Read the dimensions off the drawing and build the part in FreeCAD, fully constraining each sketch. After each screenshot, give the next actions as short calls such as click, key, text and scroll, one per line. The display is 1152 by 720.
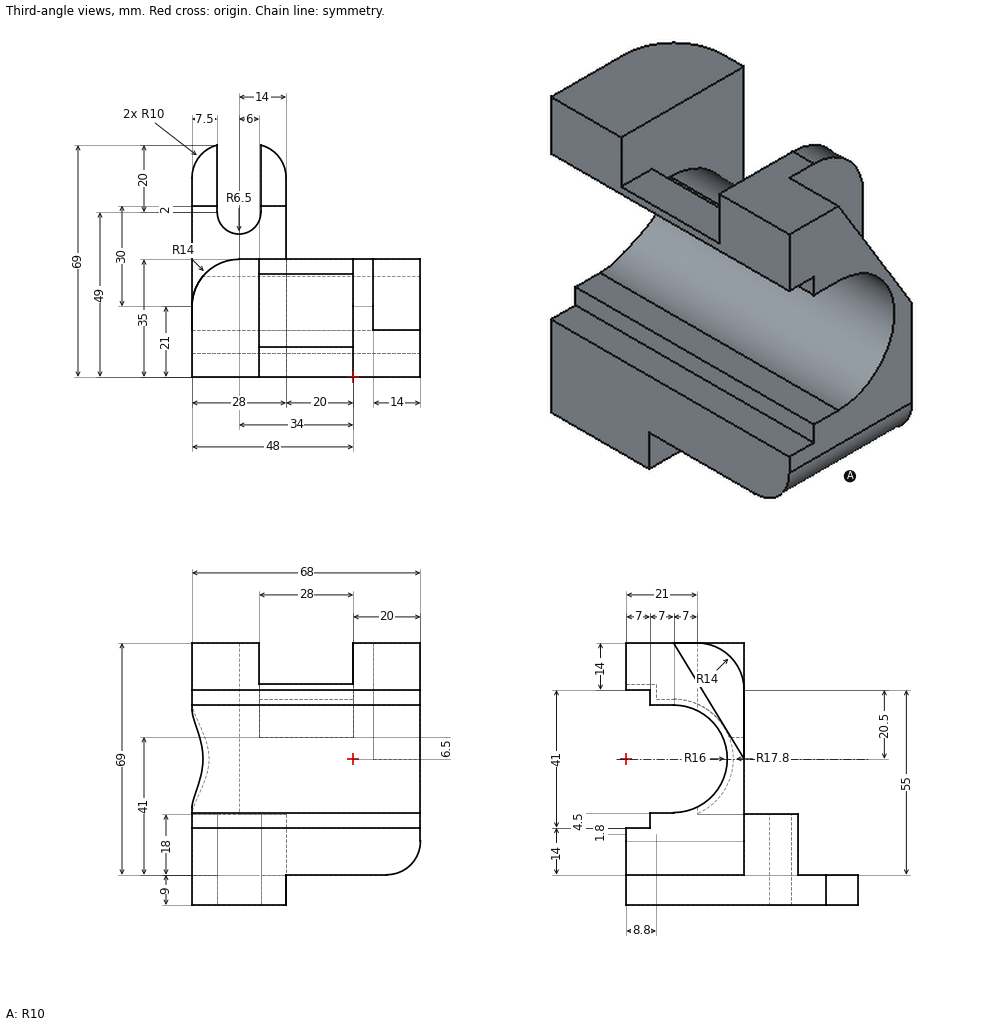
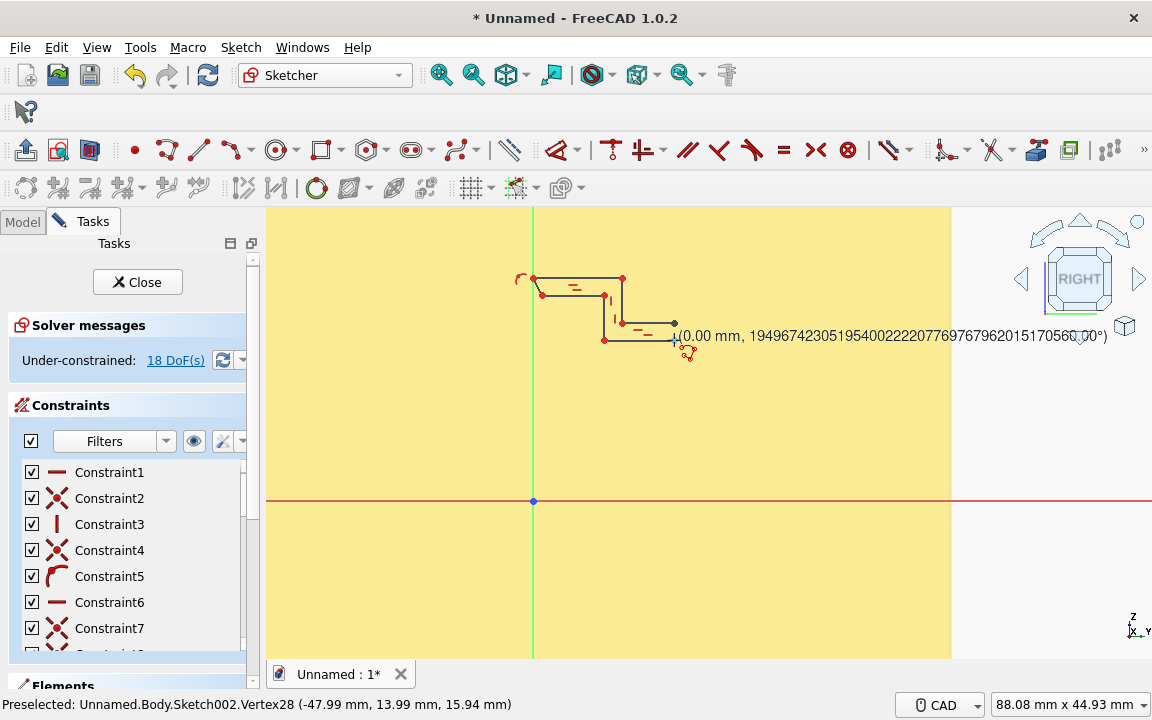
click(232, 150)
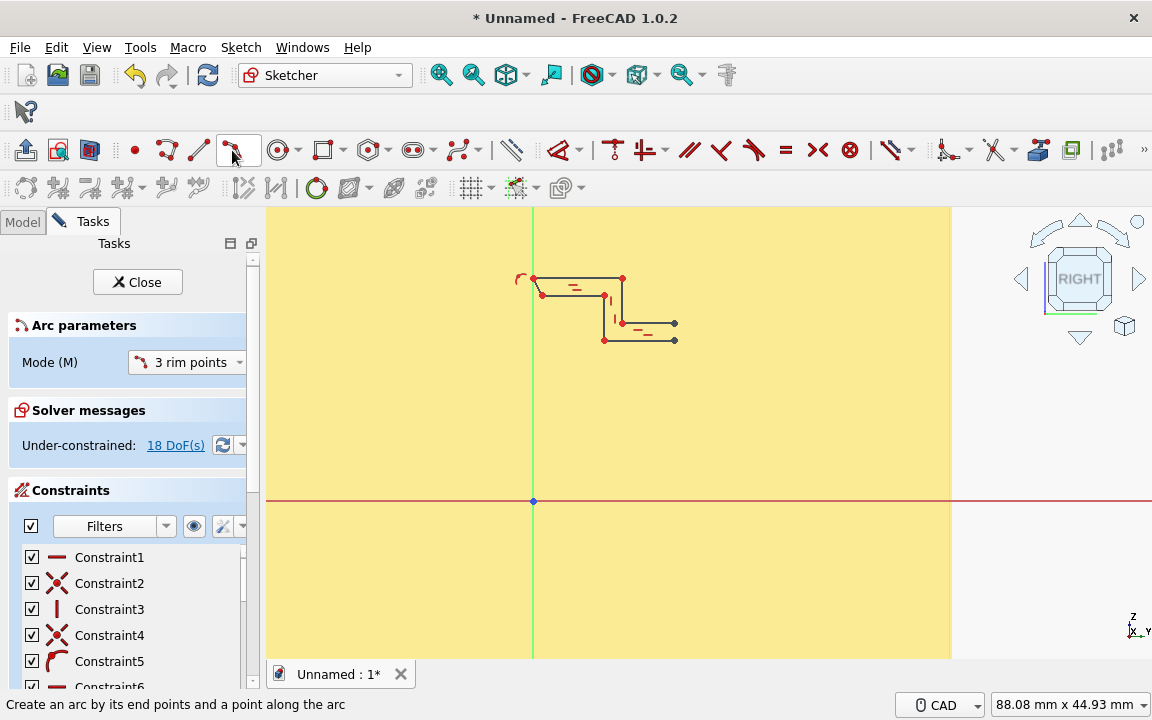
scroll(533, 294, down, 2)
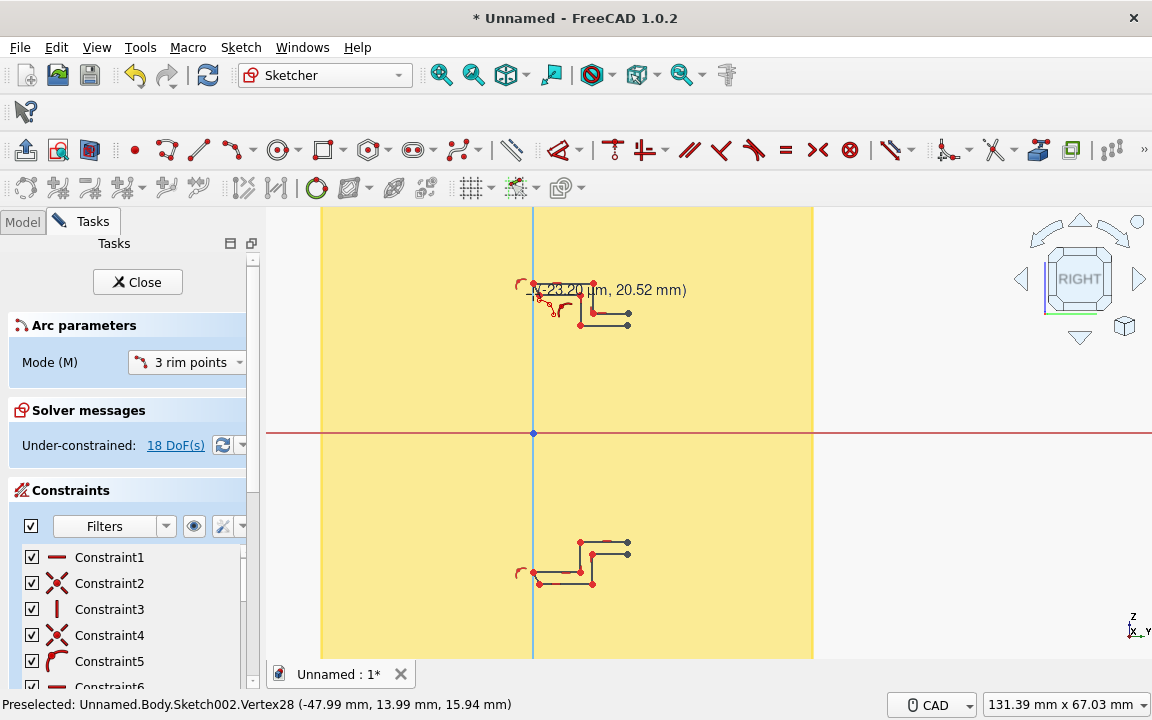
scroll(628, 553, up, 2)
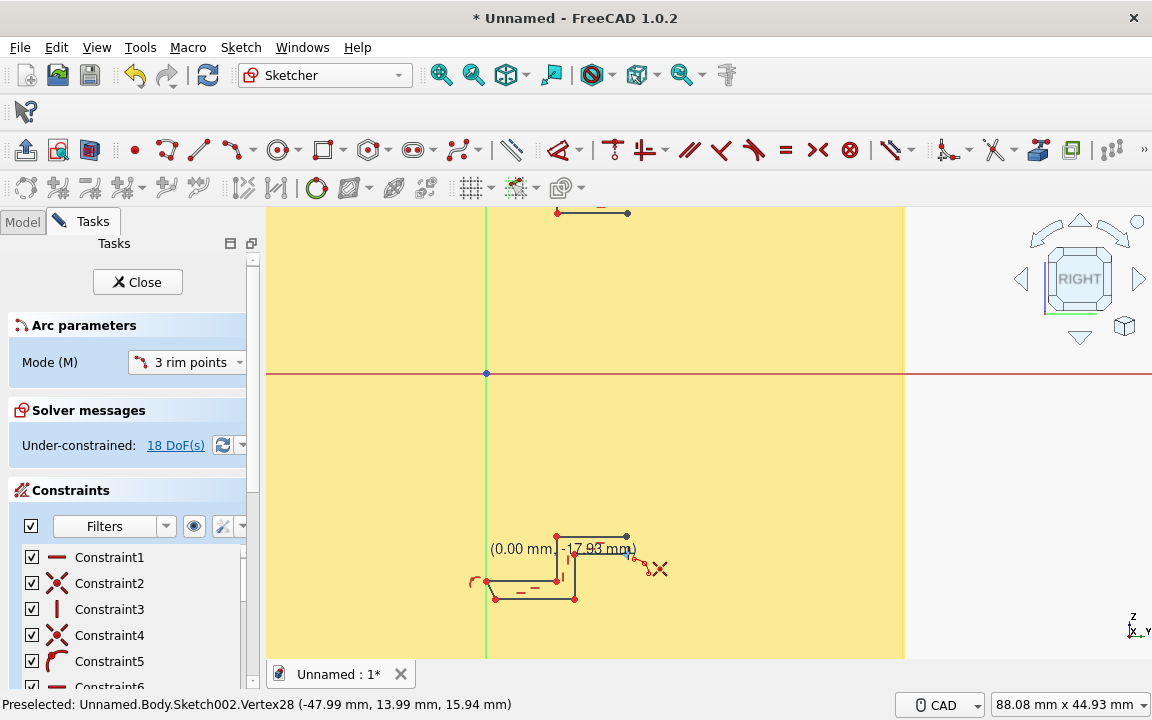
click(627, 554)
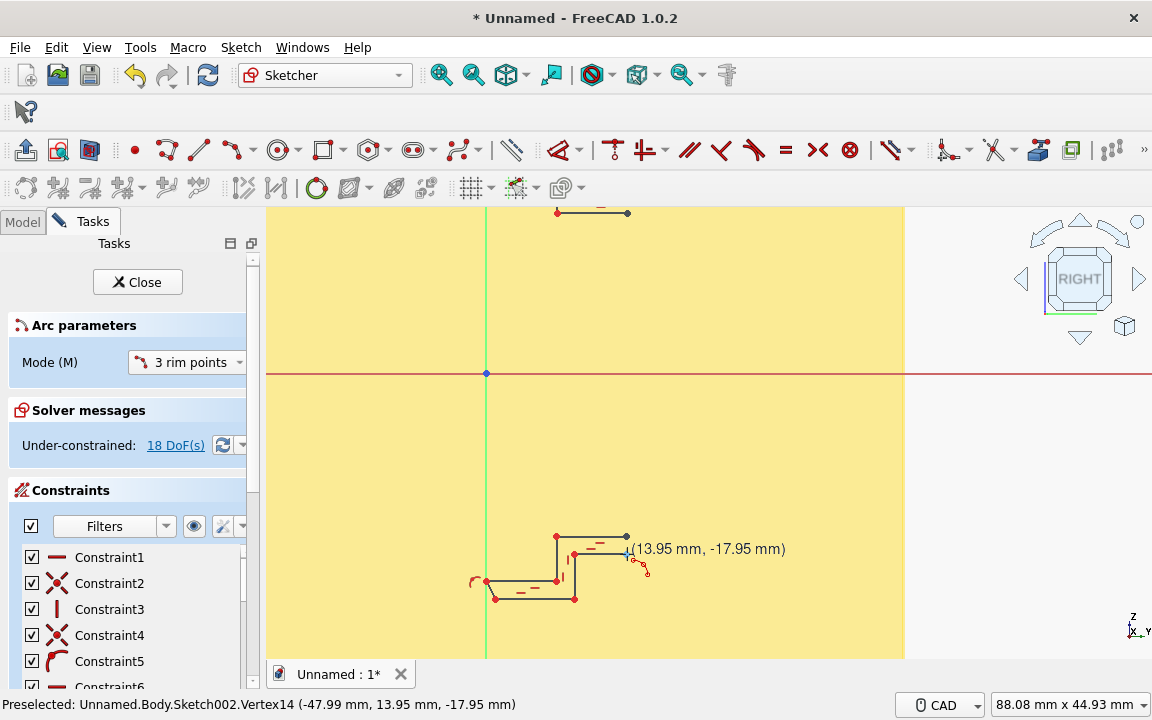
scroll(628, 554, down, 2)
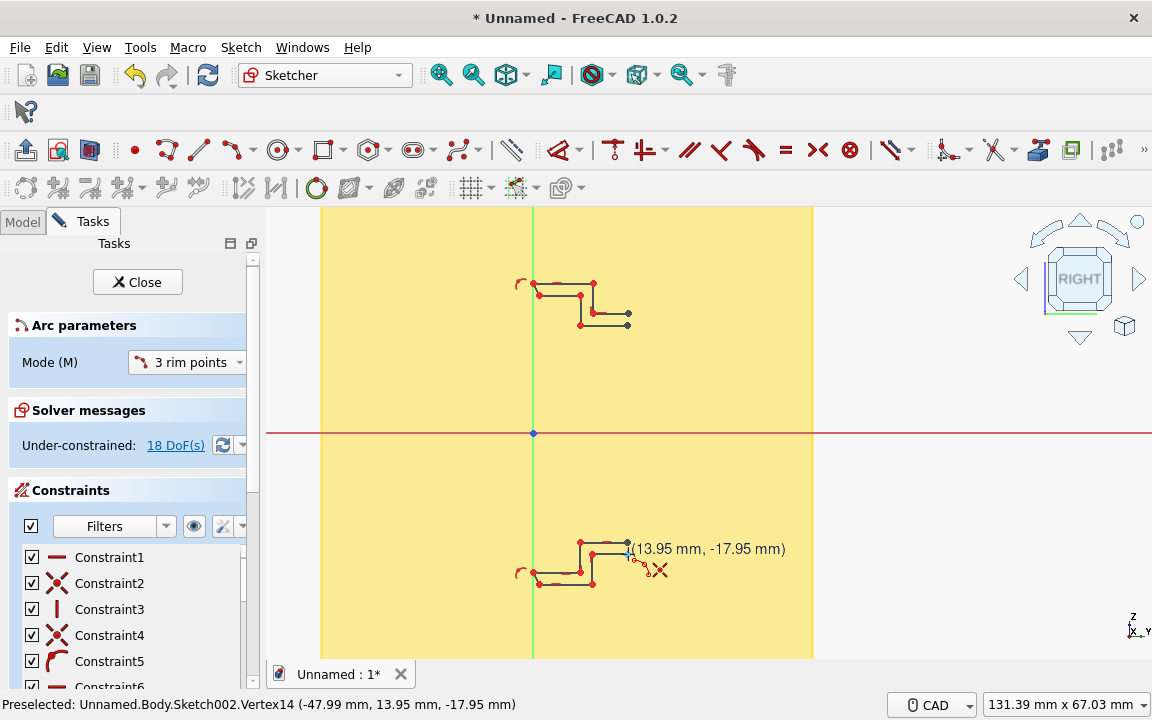
scroll(628, 313, up, 2)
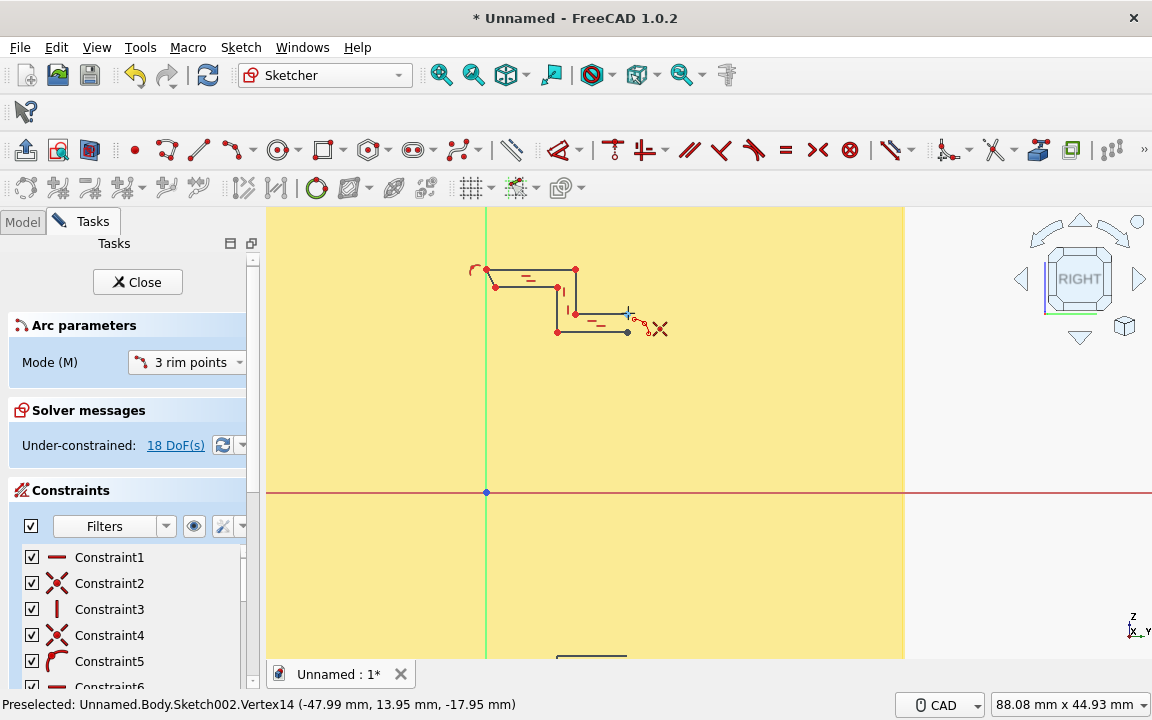
click(628, 314)
click(798, 548)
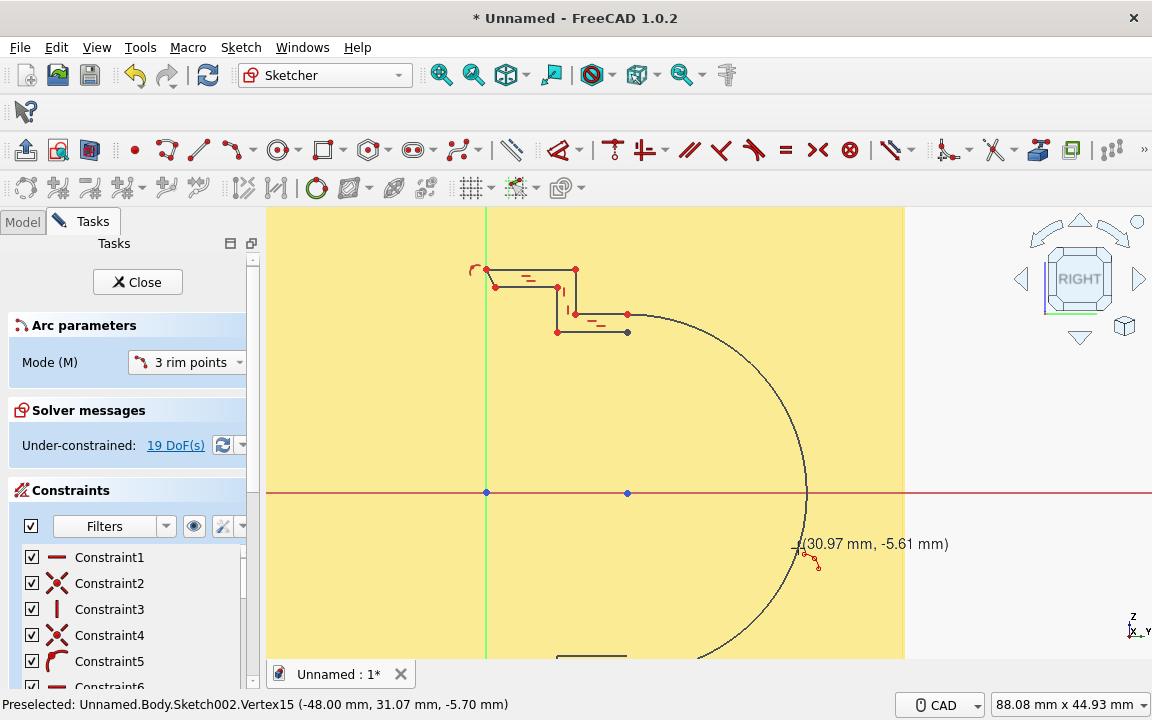
click(627, 332)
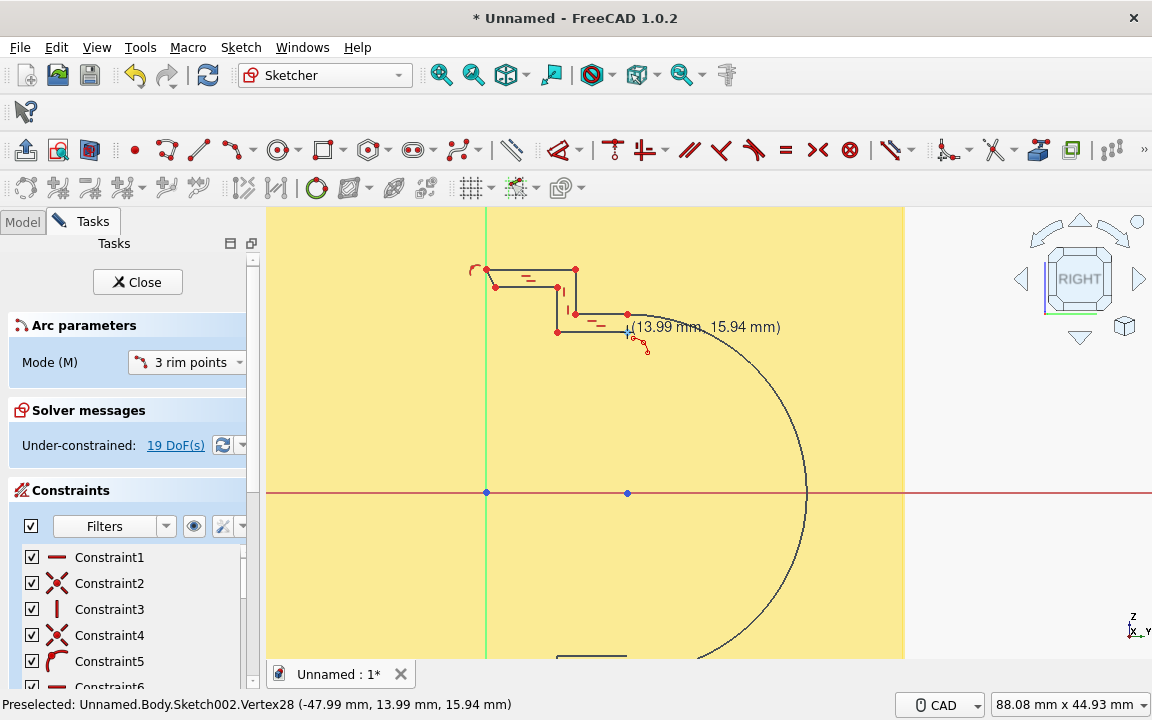
scroll(628, 312, down, 2)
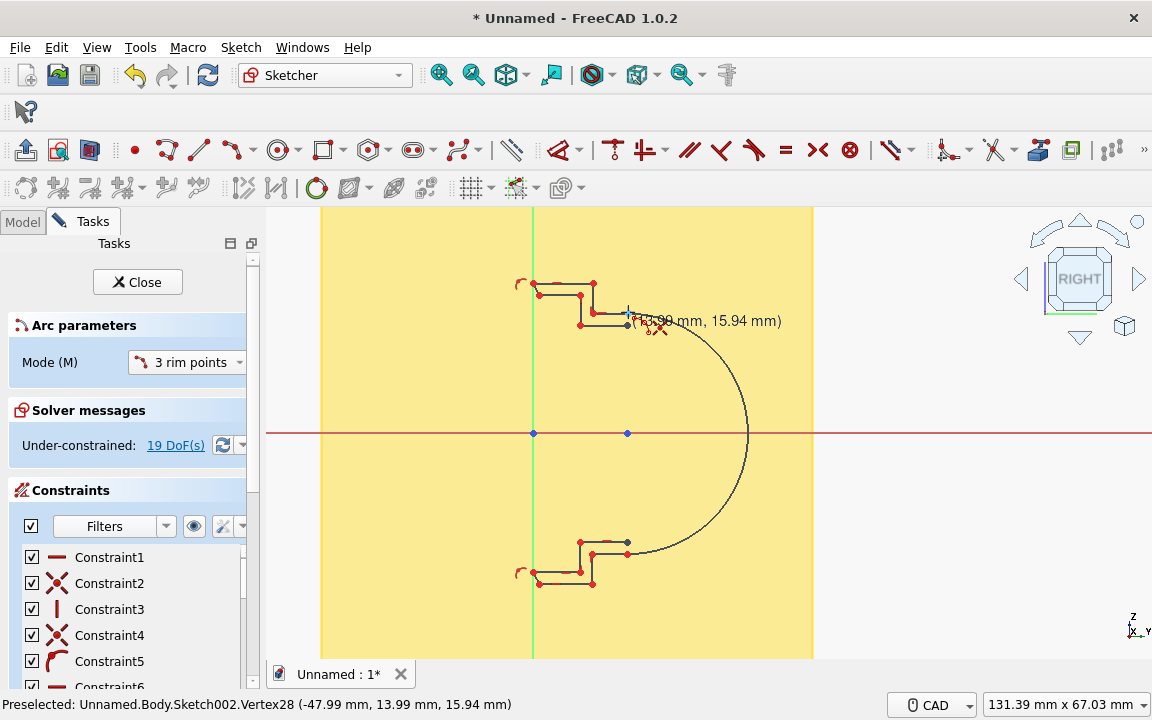
scroll(628, 541, up, 2)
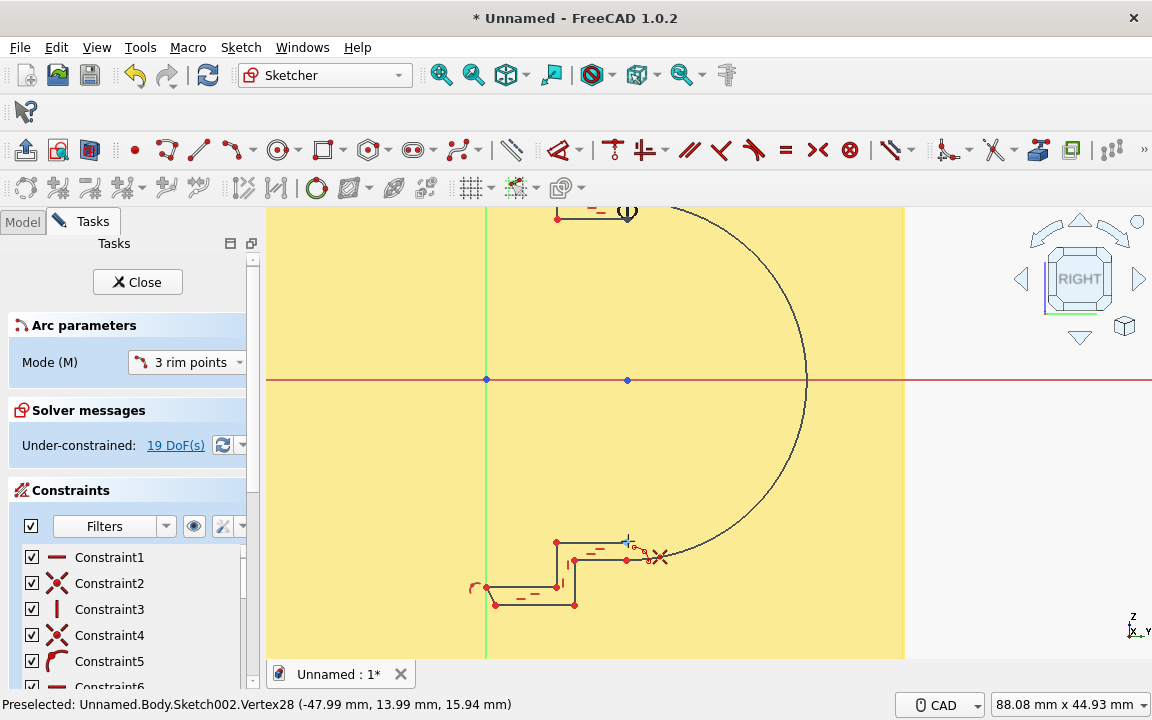
click(627, 543)
click(780, 429)
key(Escape)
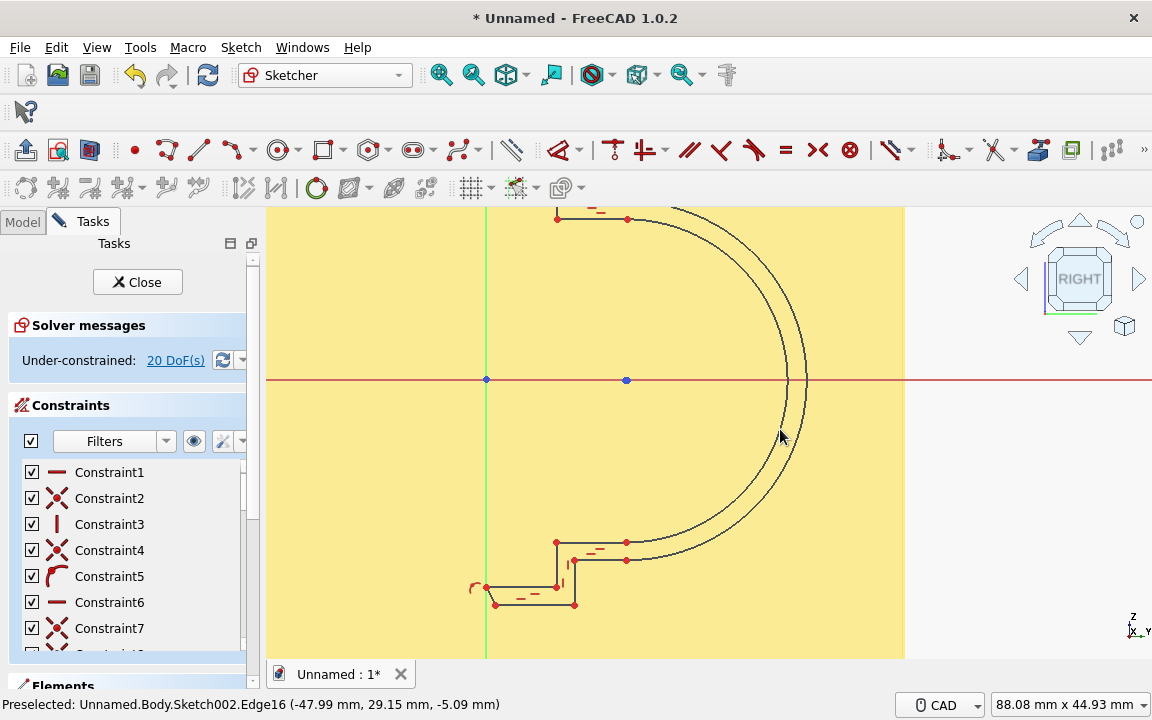
click(578, 543)